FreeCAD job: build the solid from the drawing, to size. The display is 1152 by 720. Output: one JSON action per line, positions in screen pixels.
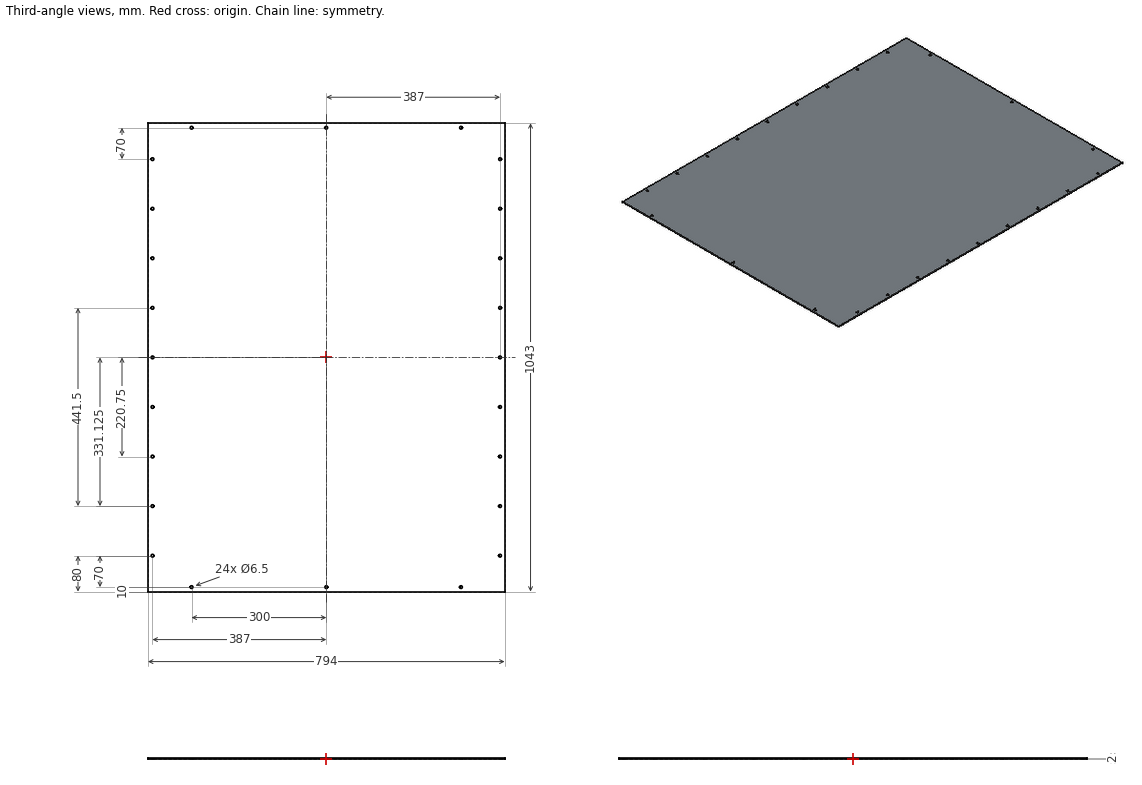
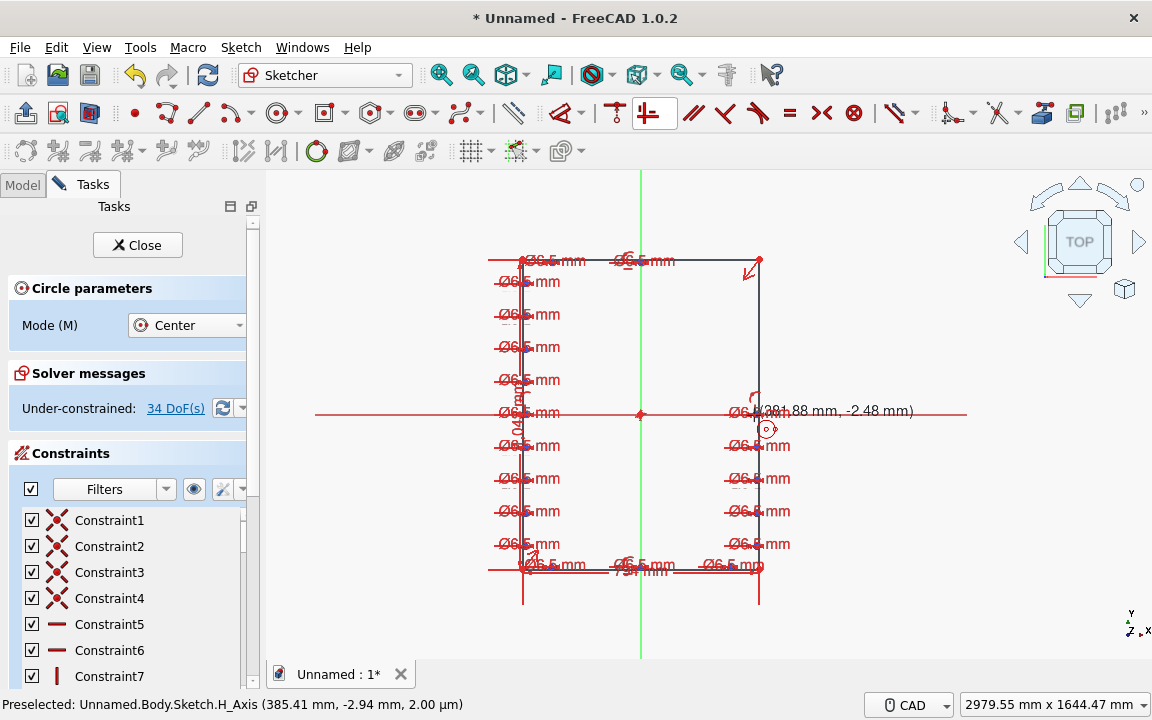
{"action": "scroll", "coordinate": [756, 382], "scroll_direction": "up", "scroll_amount": 16}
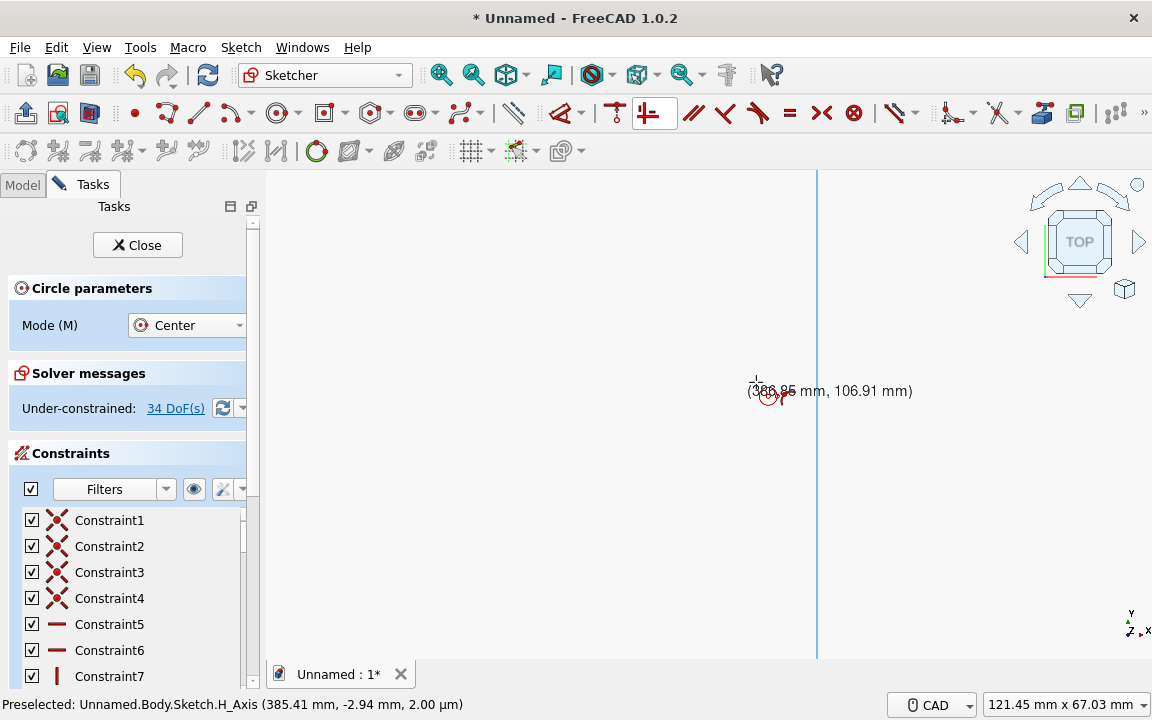
{"action": "scroll", "coordinate": [783, 375], "scroll_direction": "down", "scroll_amount": 15}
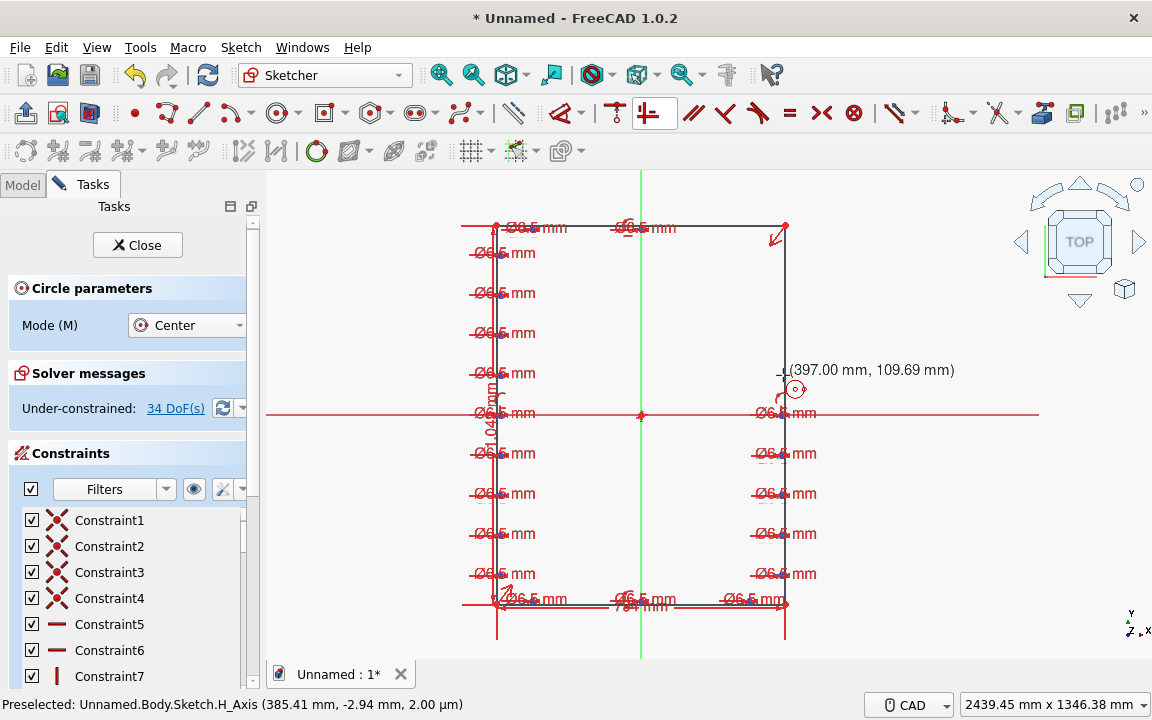
{"action": "scroll", "coordinate": [782, 375], "scroll_direction": "up", "scroll_amount": 8}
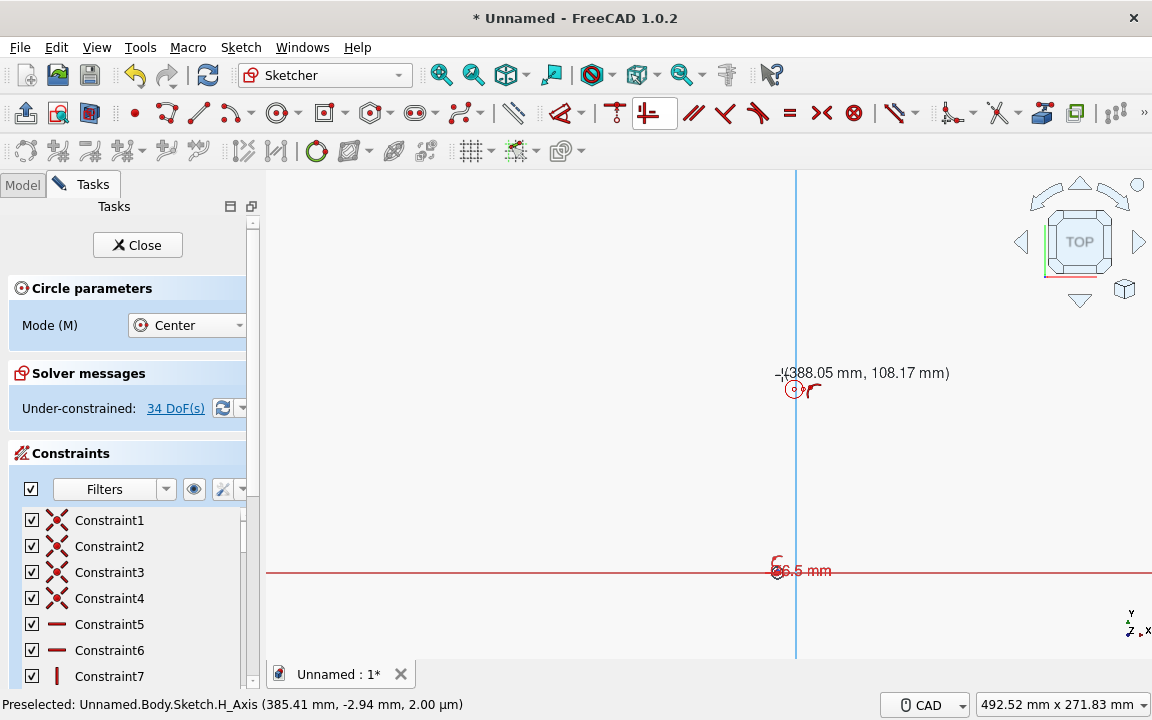
{"action": "left_click", "coordinate": [778, 374]}
{"action": "mouse_move", "coordinate": [774, 370]}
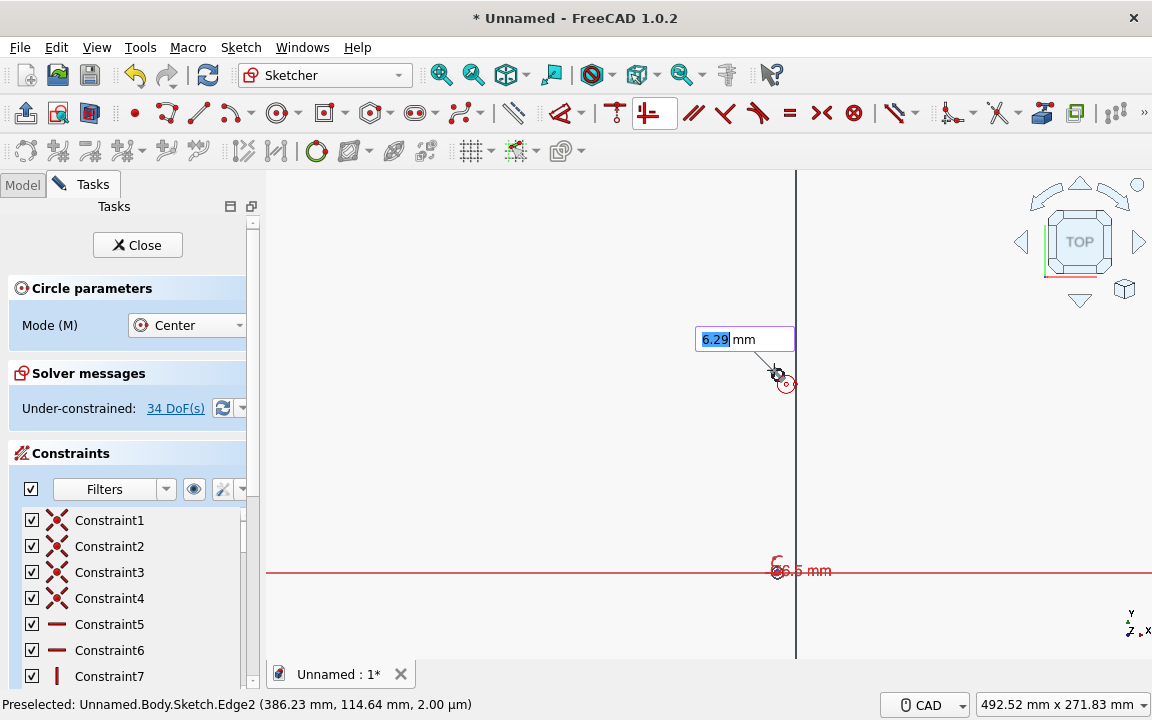
{"action": "type", "text": "6.5"}
{"action": "key", "text": "Return"}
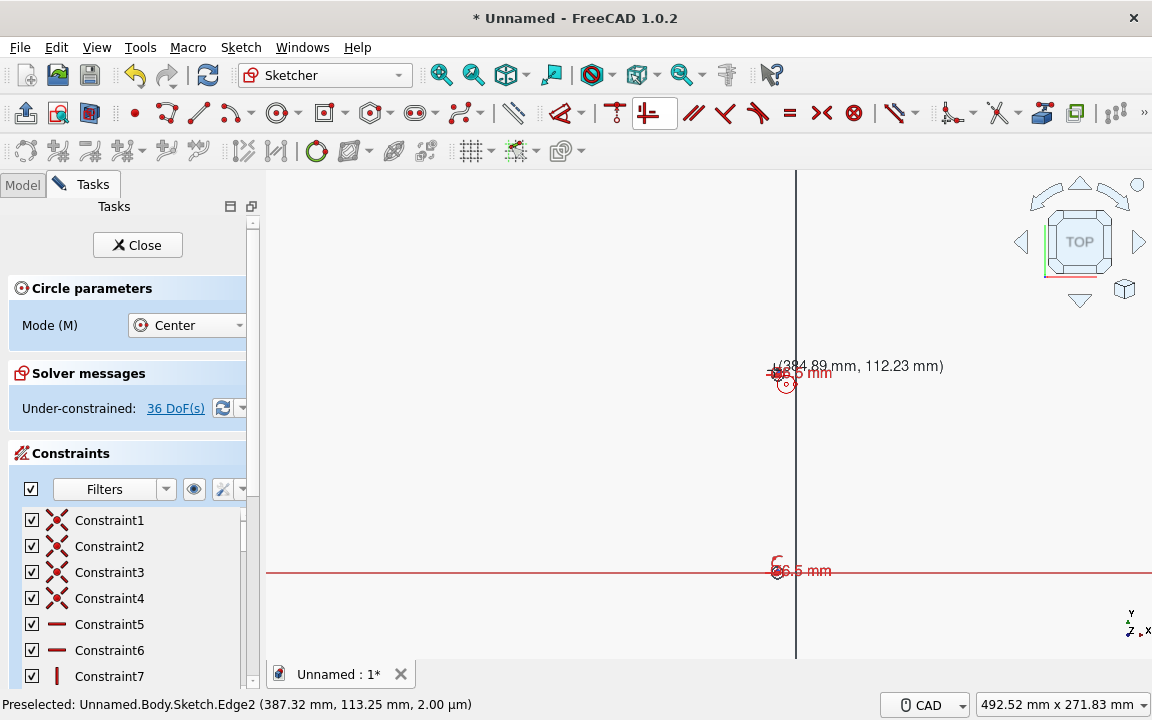
{"action": "scroll", "coordinate": [751, 383], "scroll_direction": "down", "scroll_amount": 9}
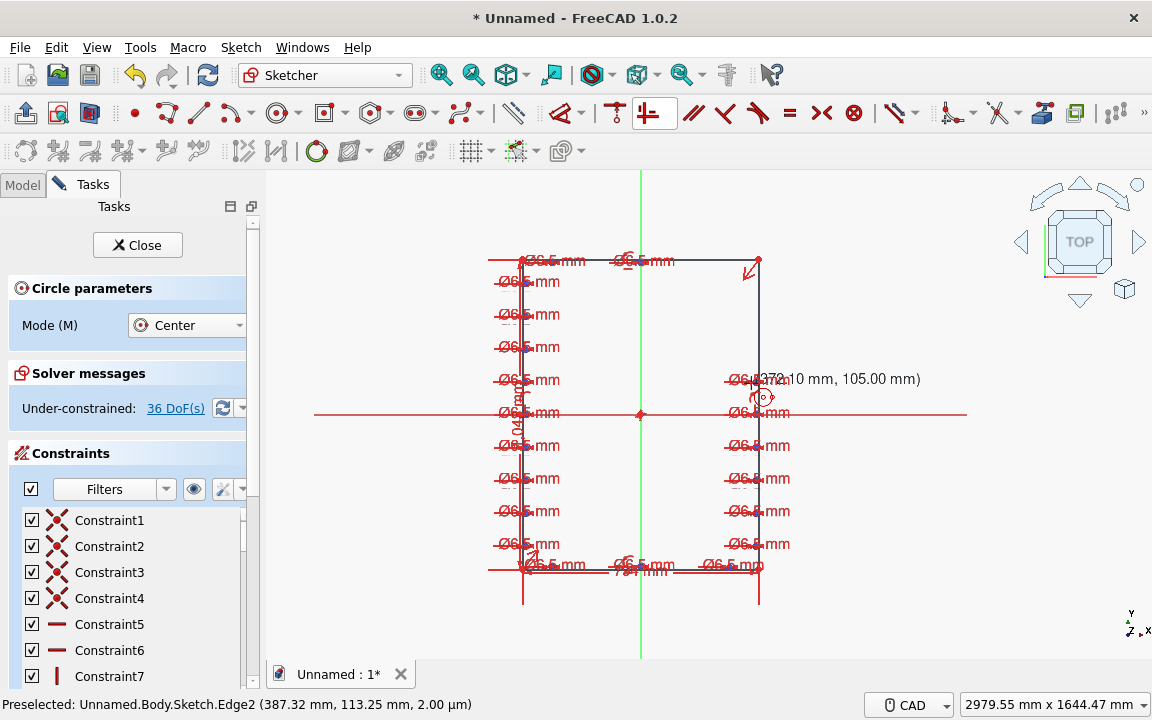
{"action": "scroll", "coordinate": [756, 349], "scroll_direction": "up", "scroll_amount": 16}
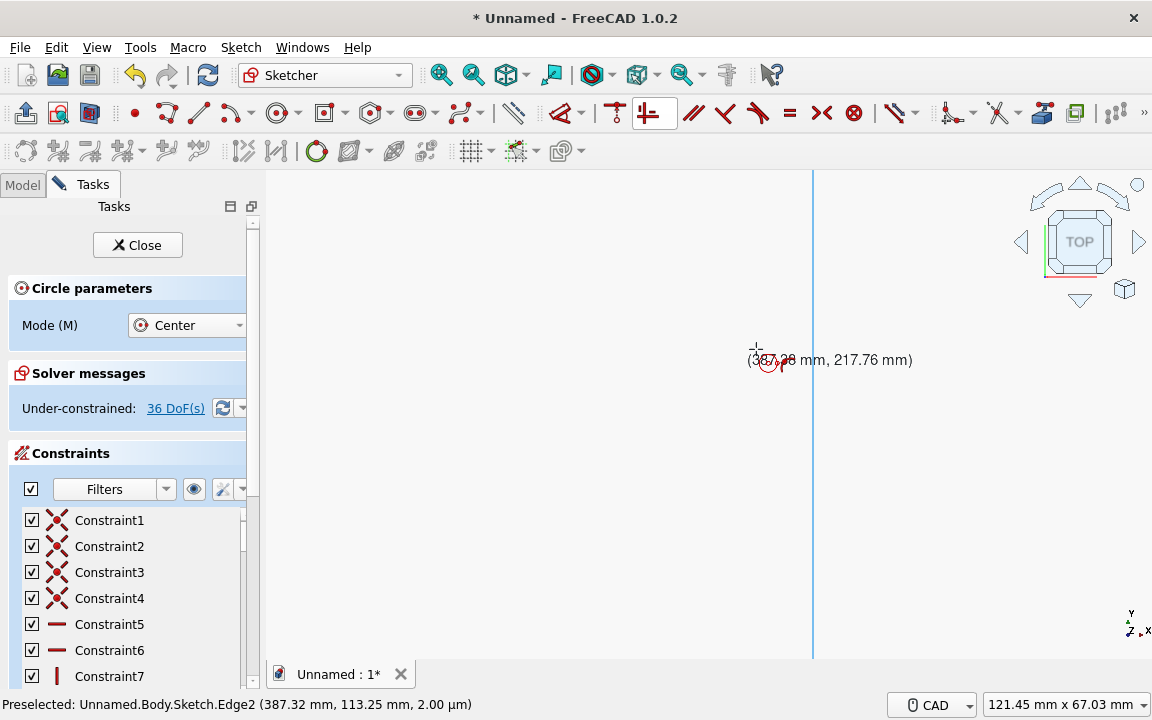
{"action": "scroll", "coordinate": [783, 334], "scroll_direction": "down", "scroll_amount": 15}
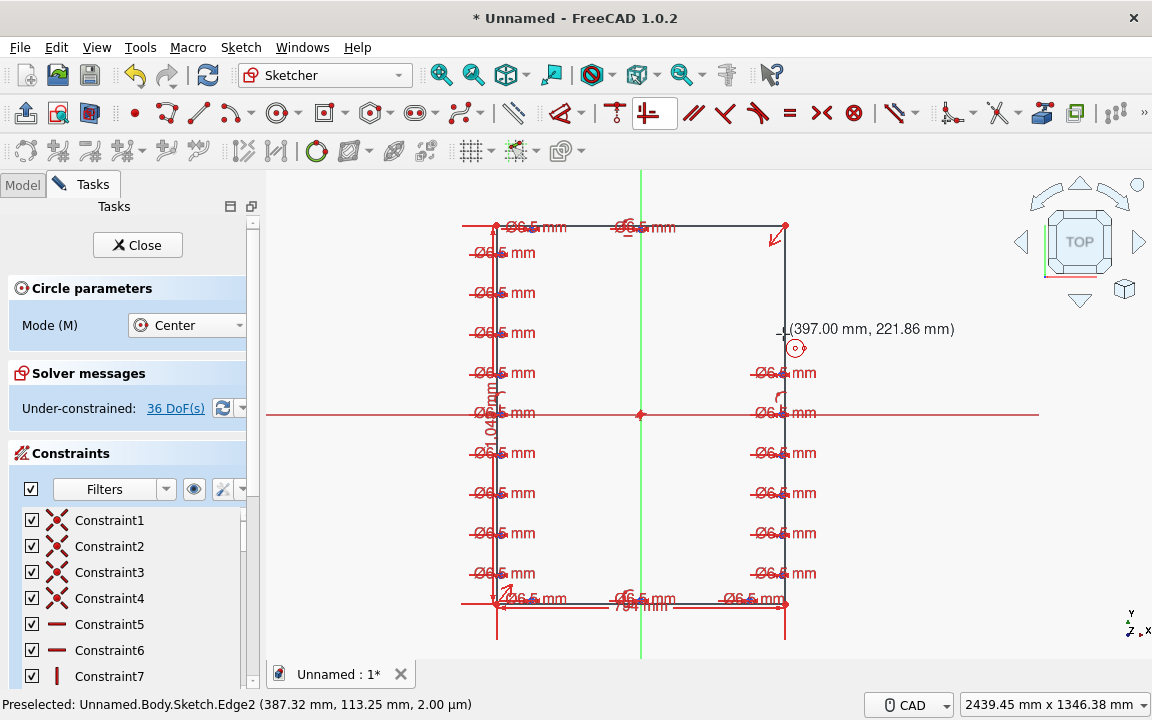
{"action": "scroll", "coordinate": [781, 335], "scroll_direction": "up", "scroll_amount": 8}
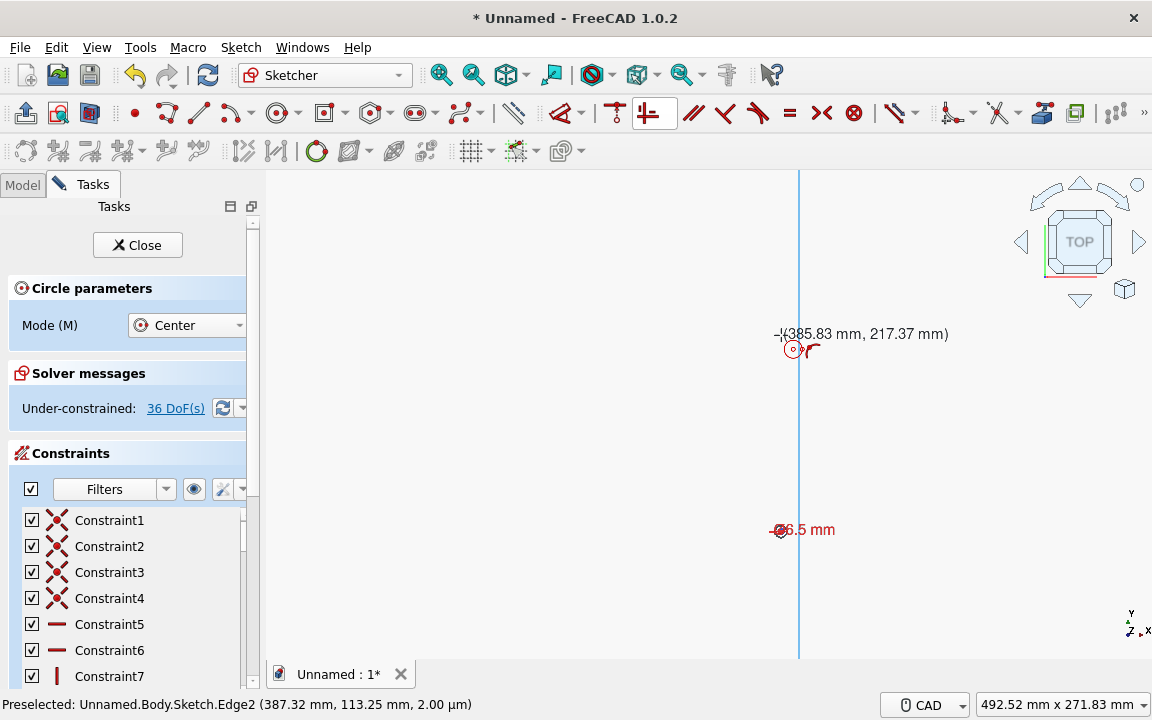
{"action": "left_click", "coordinate": [781, 333]}
{"action": "mouse_move", "coordinate": [777, 328]}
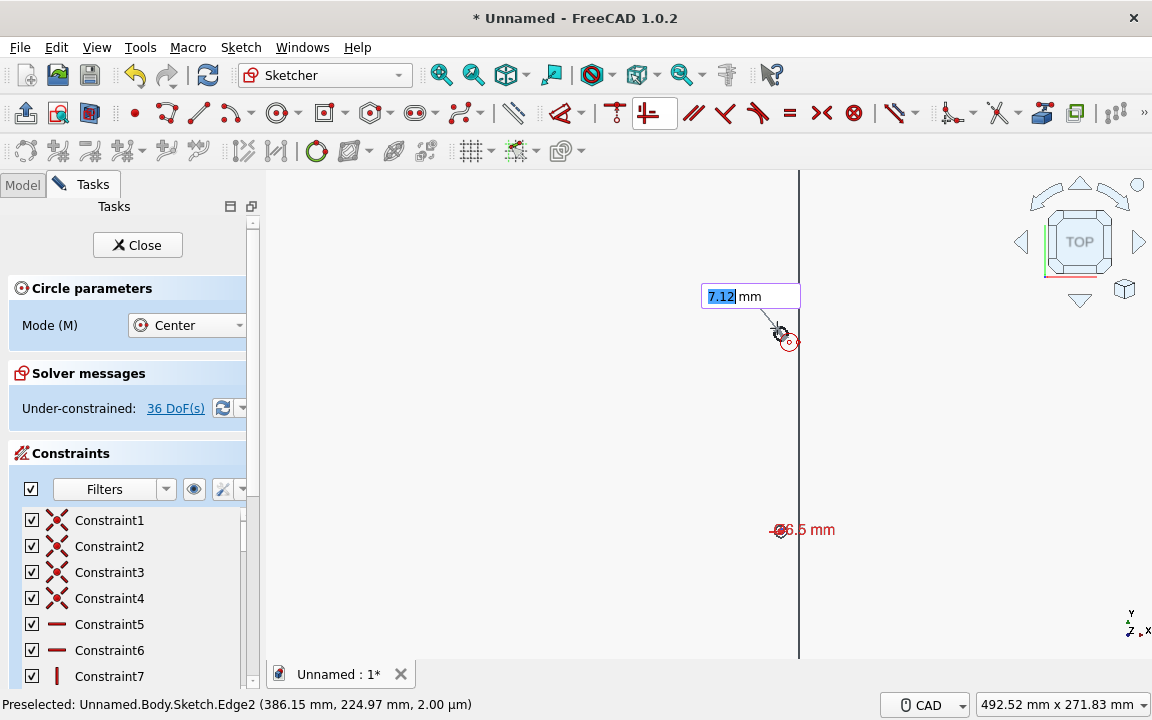
{"action": "type", "text": "6.5"}
{"action": "key", "text": "Return"}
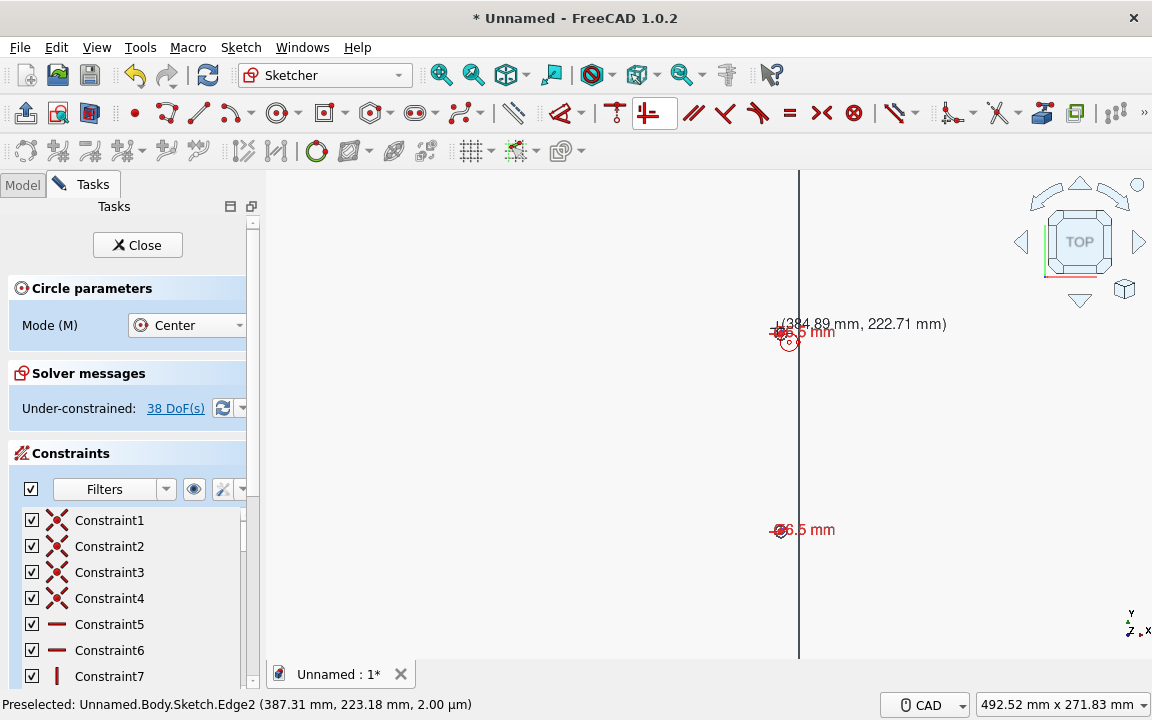
{"action": "scroll", "coordinate": [751, 352], "scroll_direction": "down", "scroll_amount": 9}